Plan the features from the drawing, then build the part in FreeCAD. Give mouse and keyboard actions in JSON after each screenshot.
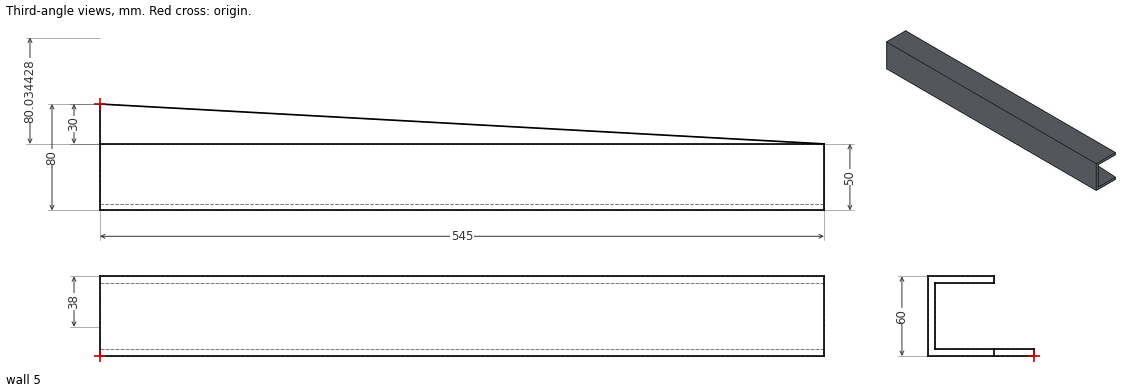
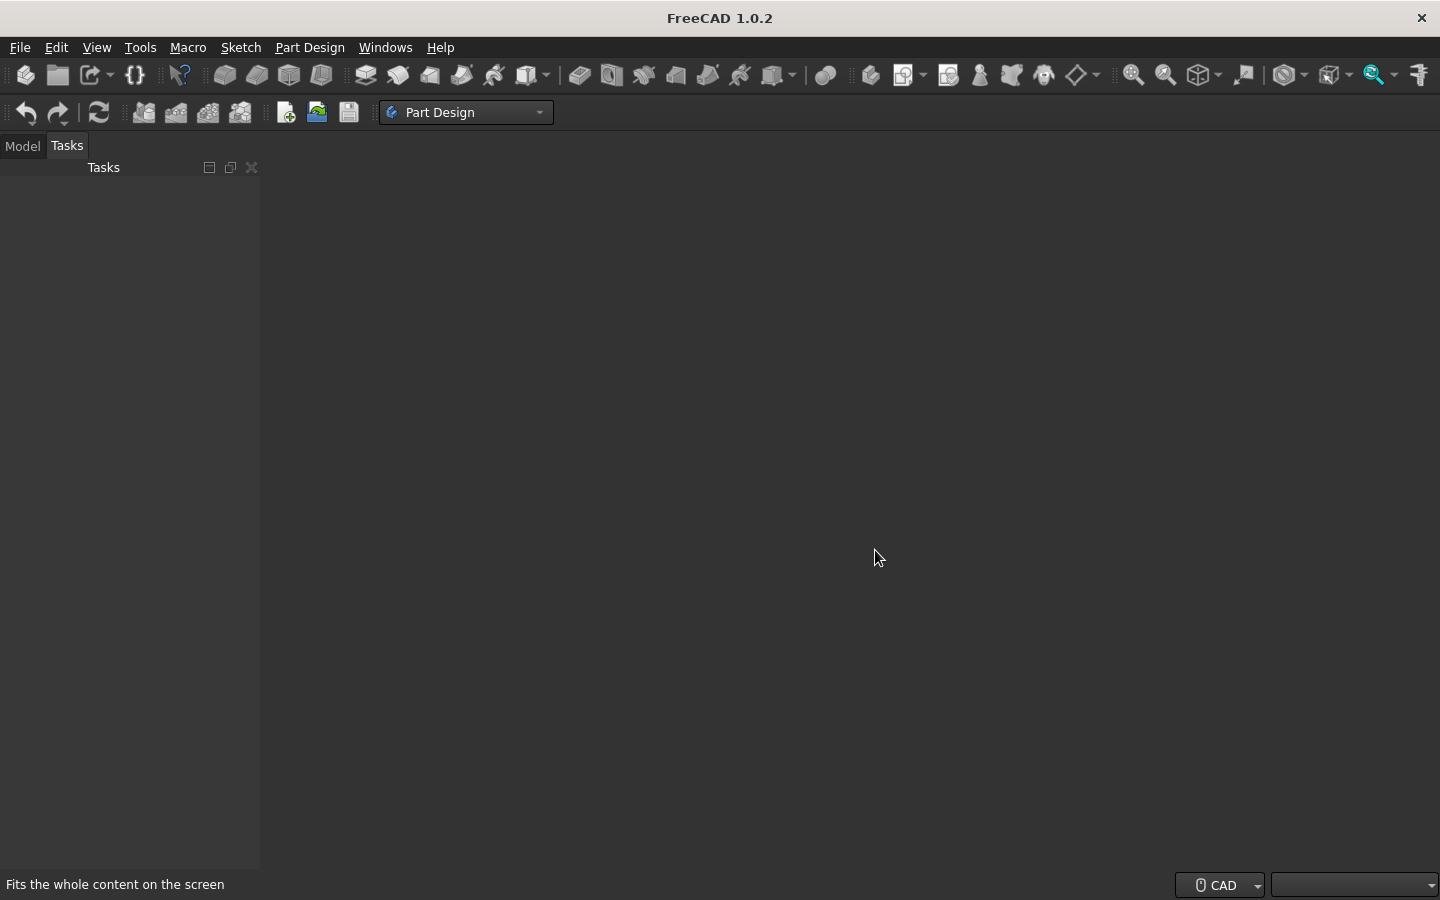
{"action": "key", "text": "ctrl+n"}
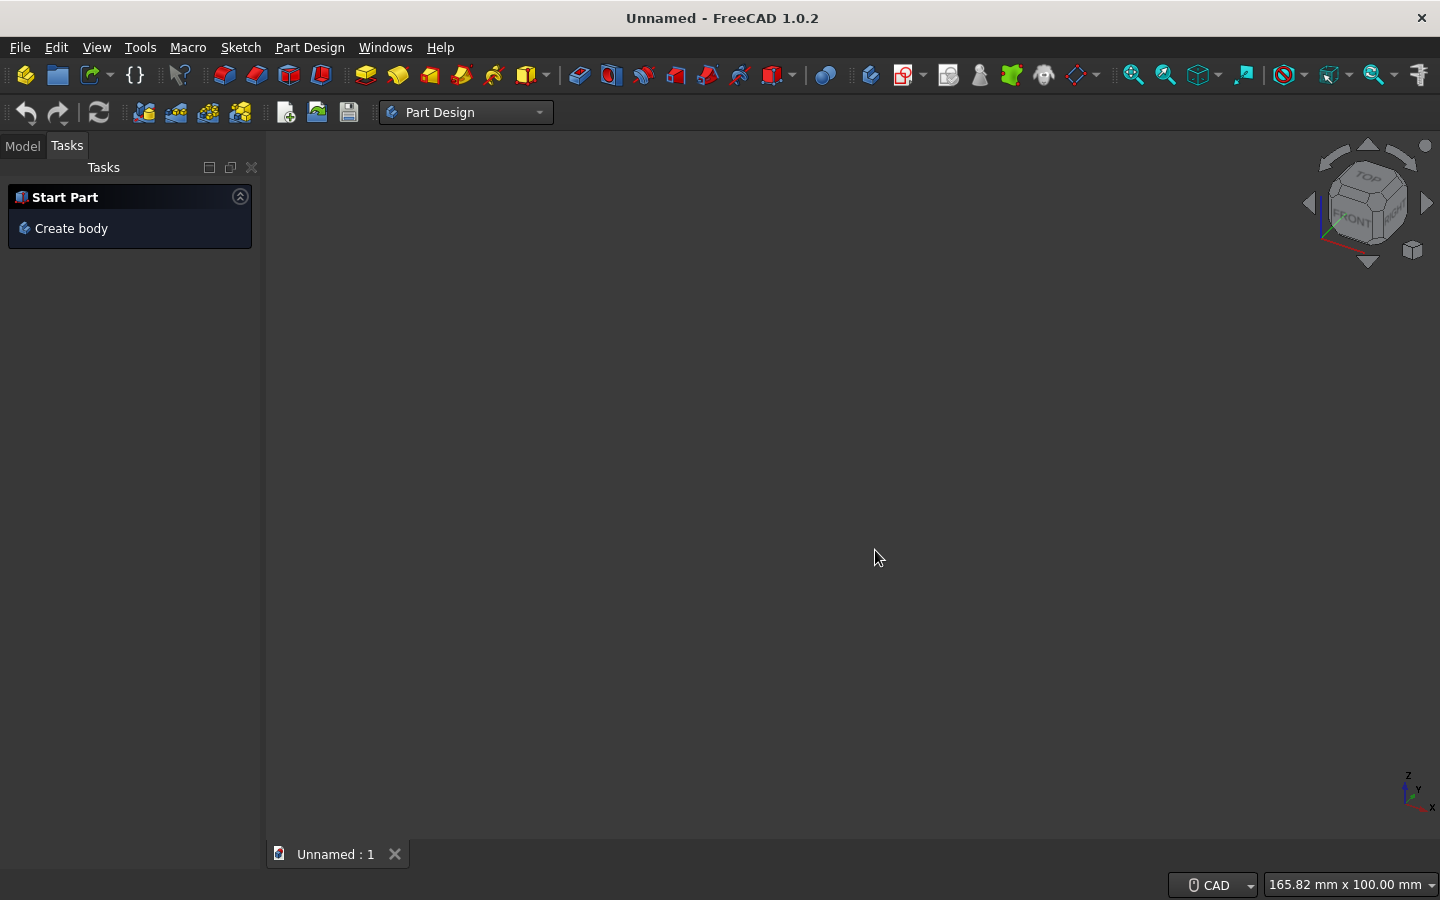
{"action": "left_click", "coordinate": [904, 76]}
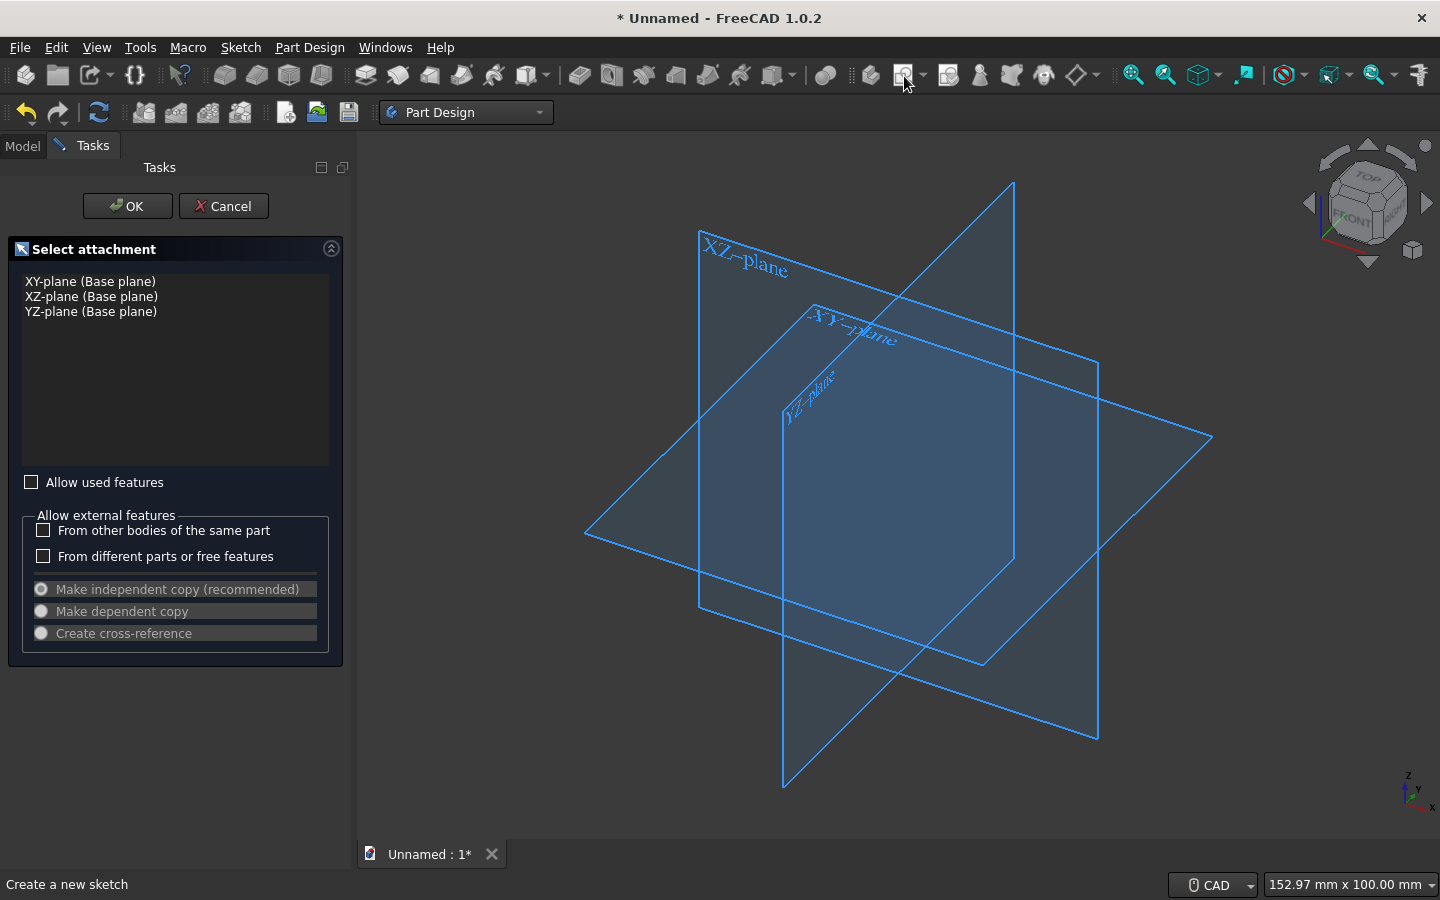
{"action": "left_click", "coordinate": [82, 282]}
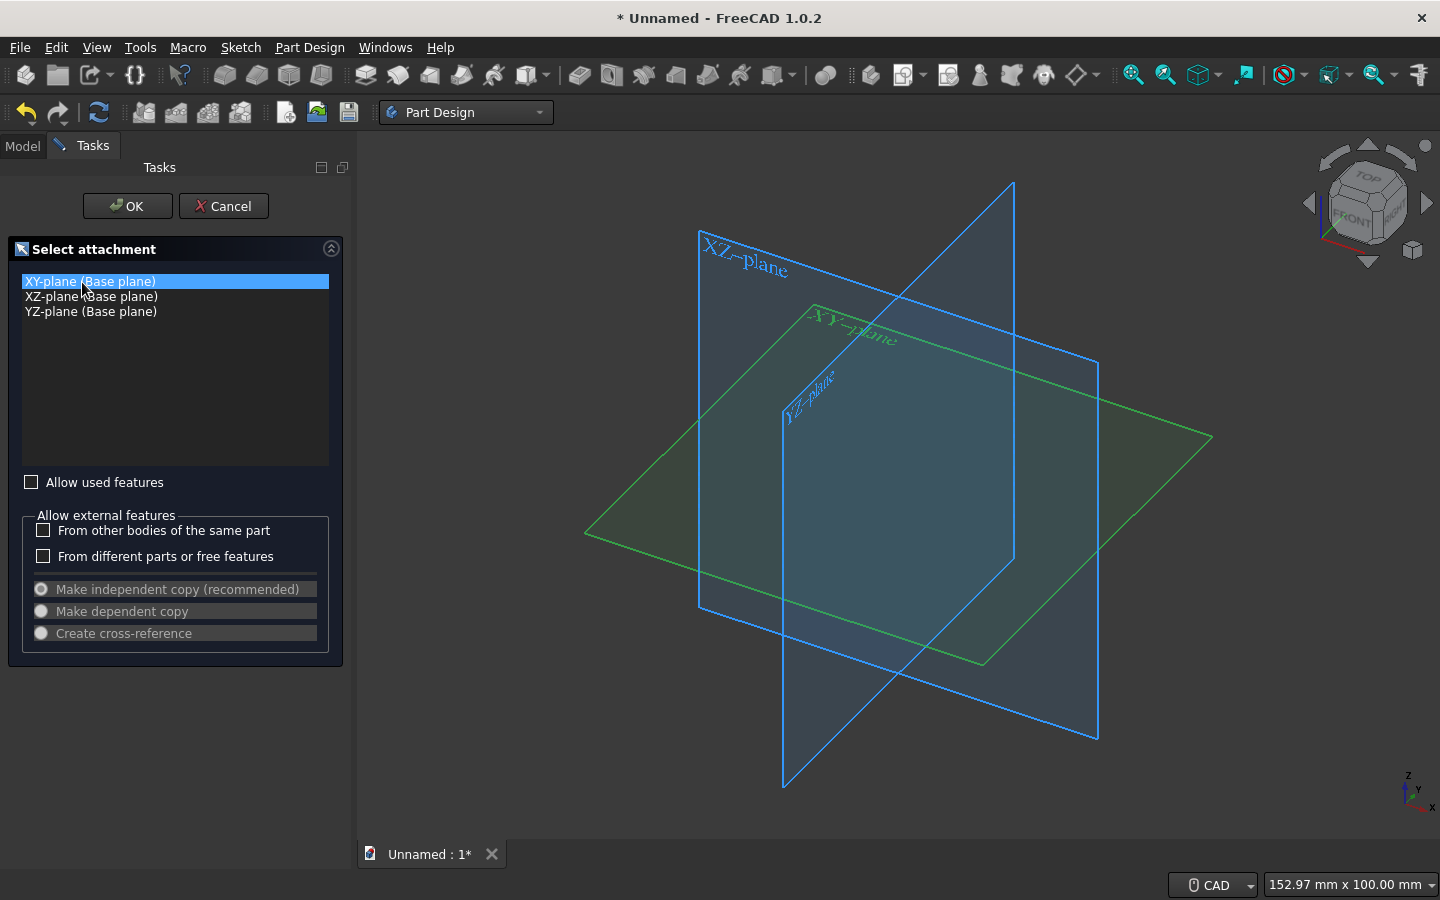
{"action": "left_click", "coordinate": [128, 206]}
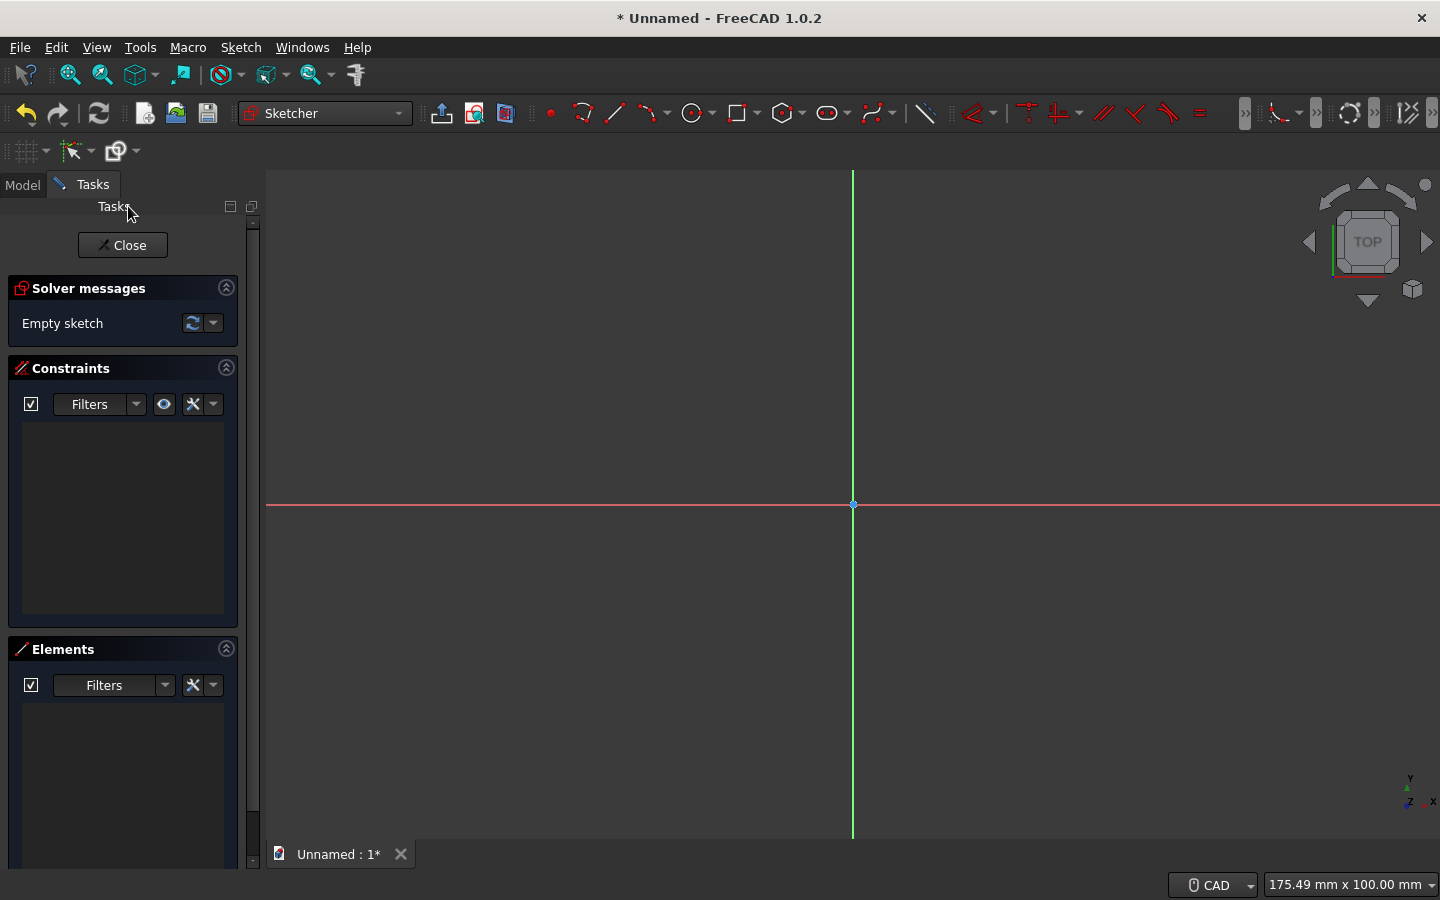
{"action": "scroll", "coordinate": [306, 437], "scroll_direction": "down", "scroll_amount": 8}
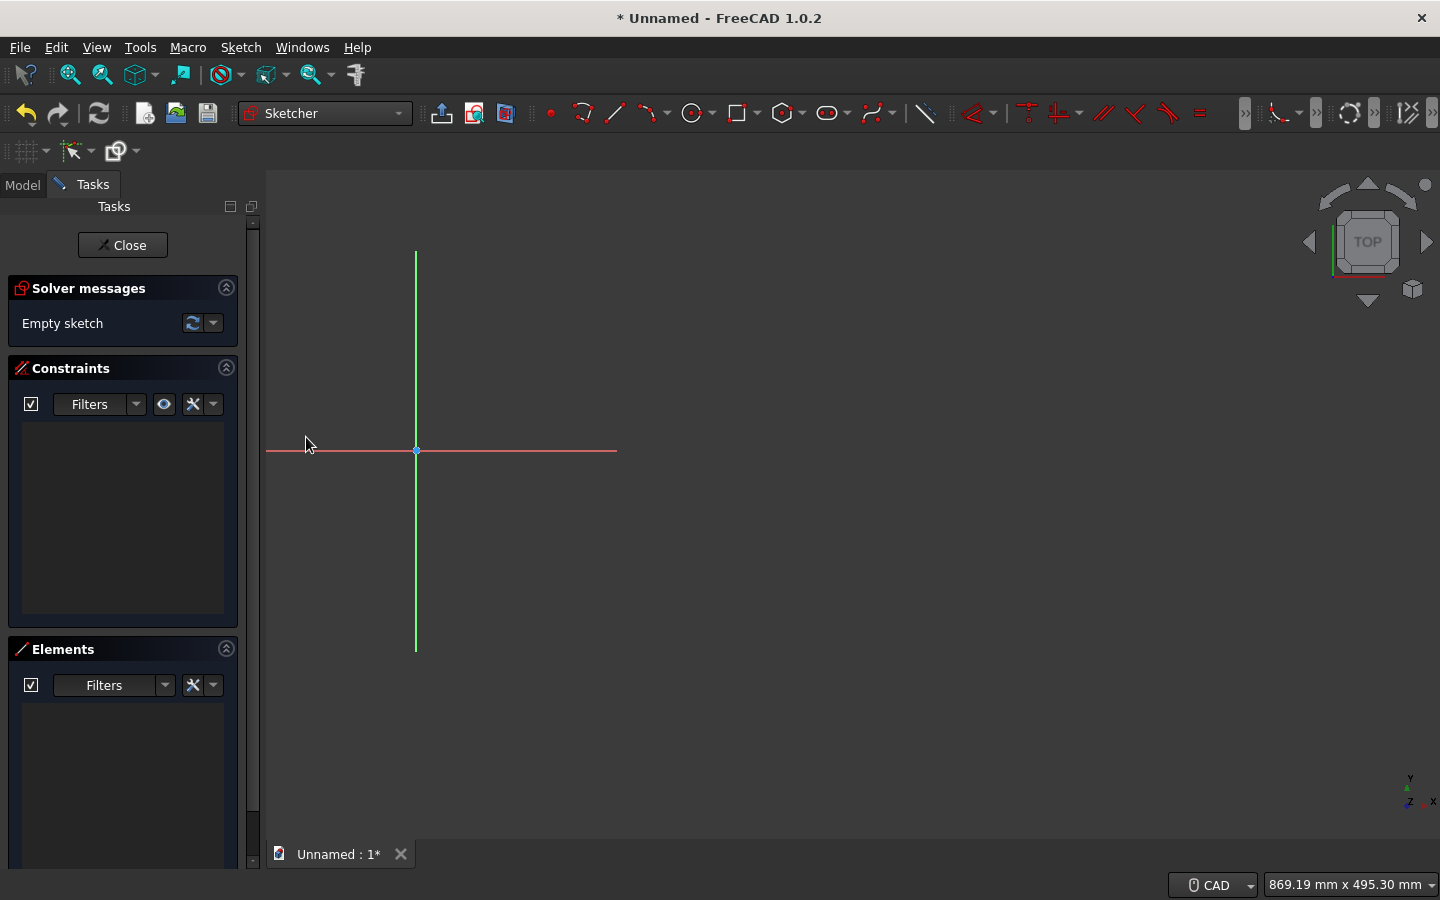
{"action": "key", "text": "g m"}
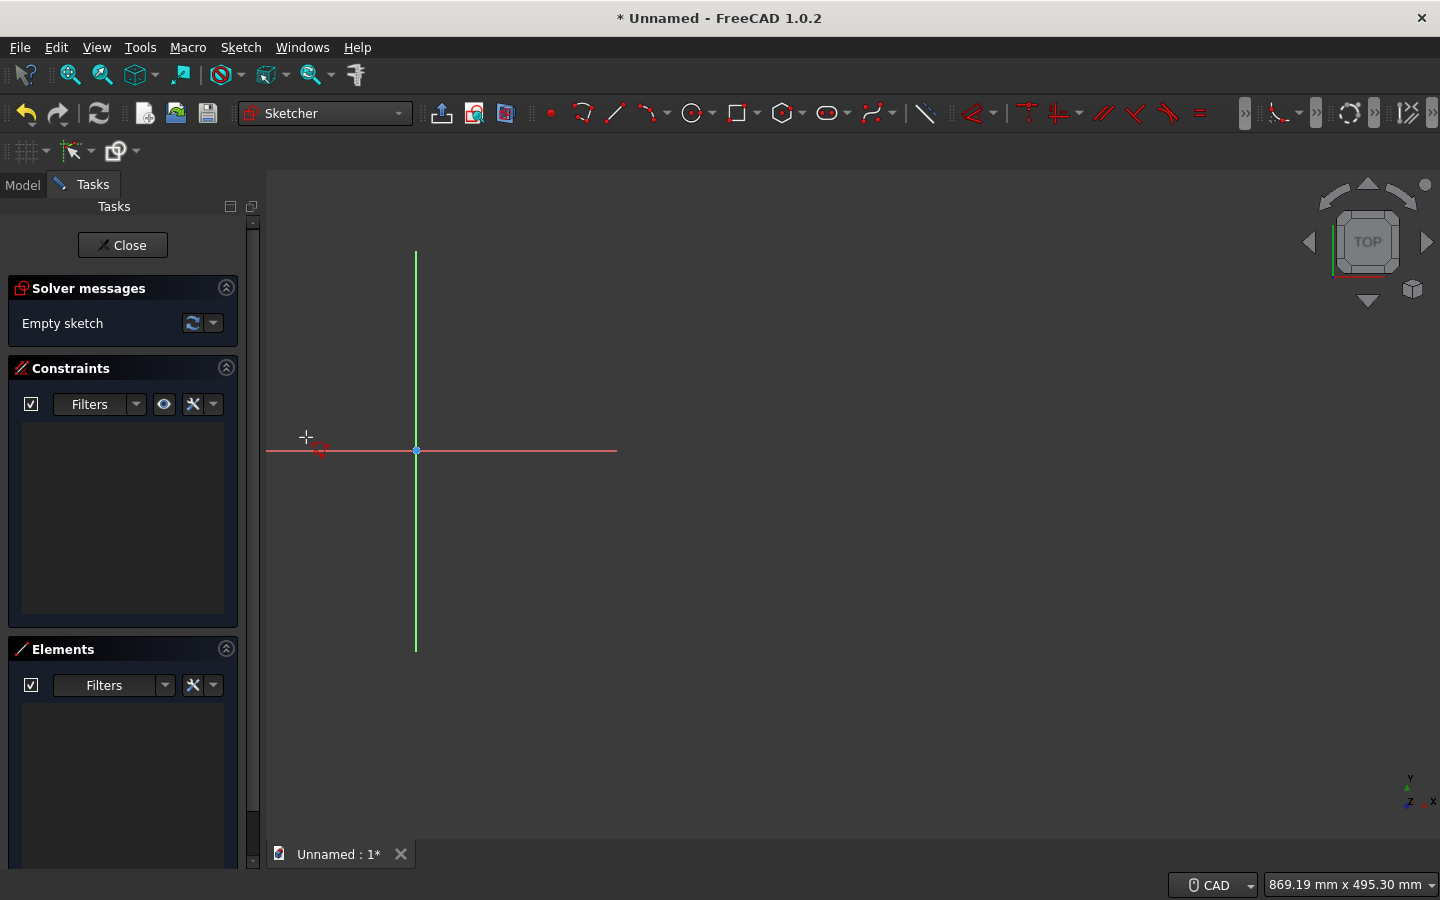
{"action": "left_click", "coordinate": [416, 451]}
{"action": "left_click", "coordinate": [425, 559]}
{"action": "left_click", "coordinate": [1153, 559]}
{"action": "left_click", "coordinate": [1153, 491]}
{"action": "left_click", "coordinate": [416, 451]}
{"action": "key", "text": "Escape"}
{"action": "key", "text": "Escape"}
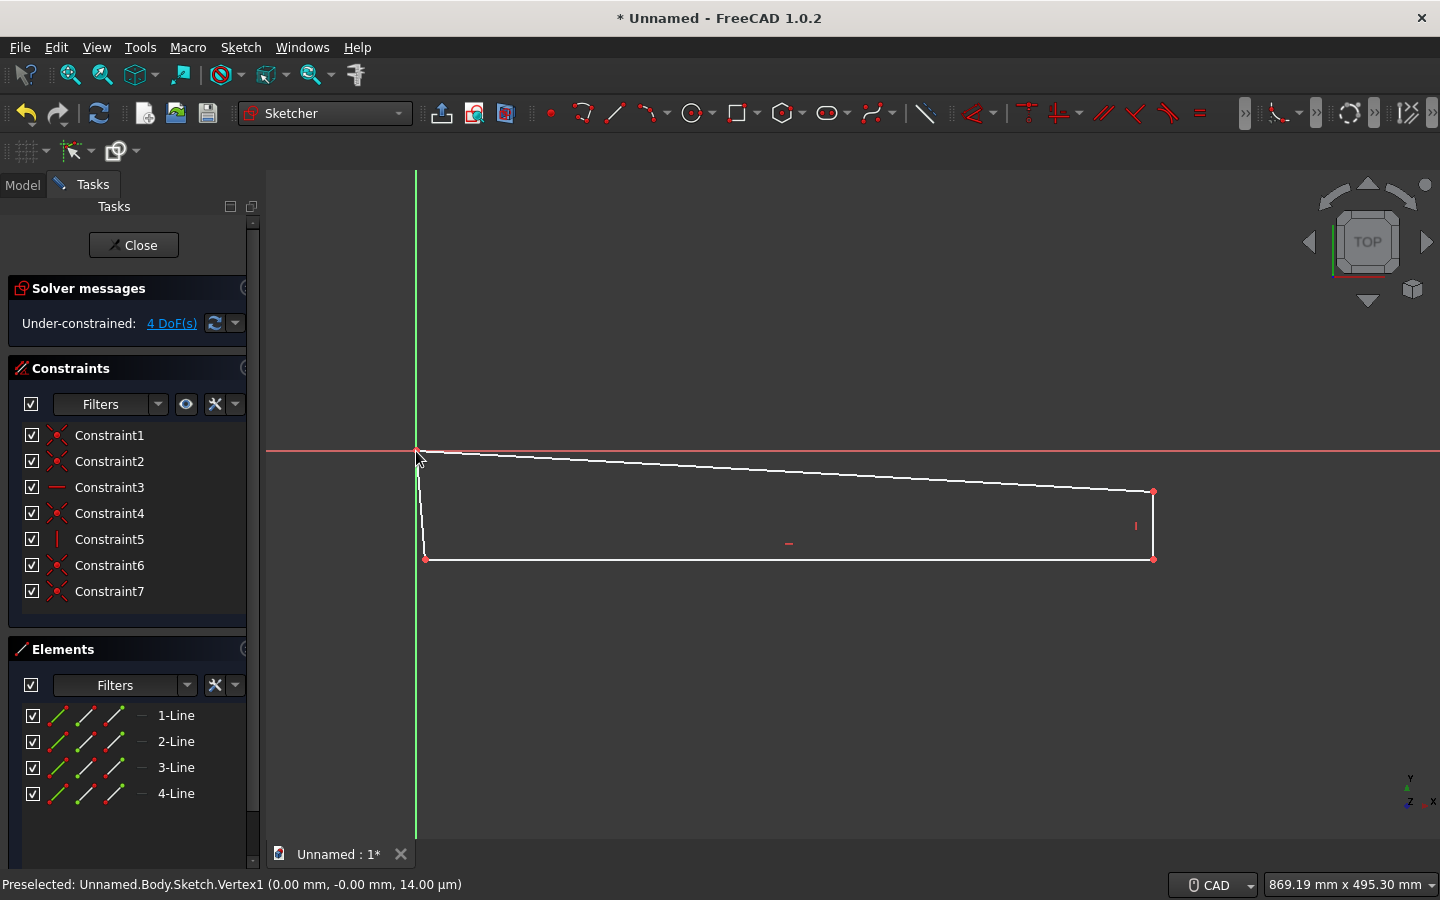
{"action": "left_click", "coordinate": [419, 484]}